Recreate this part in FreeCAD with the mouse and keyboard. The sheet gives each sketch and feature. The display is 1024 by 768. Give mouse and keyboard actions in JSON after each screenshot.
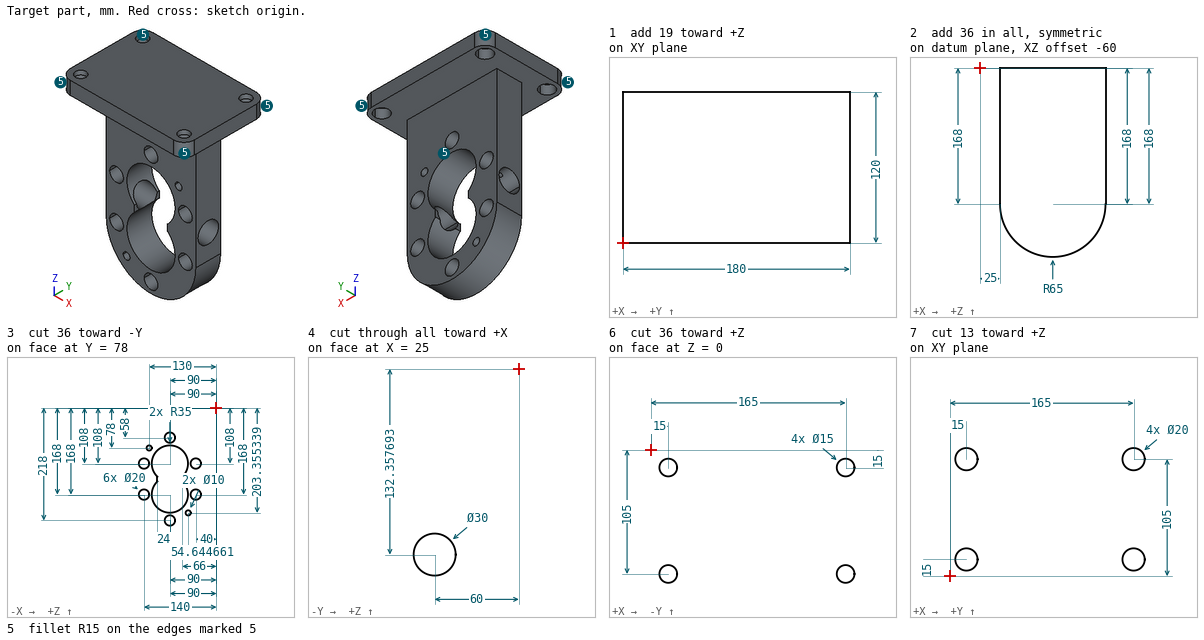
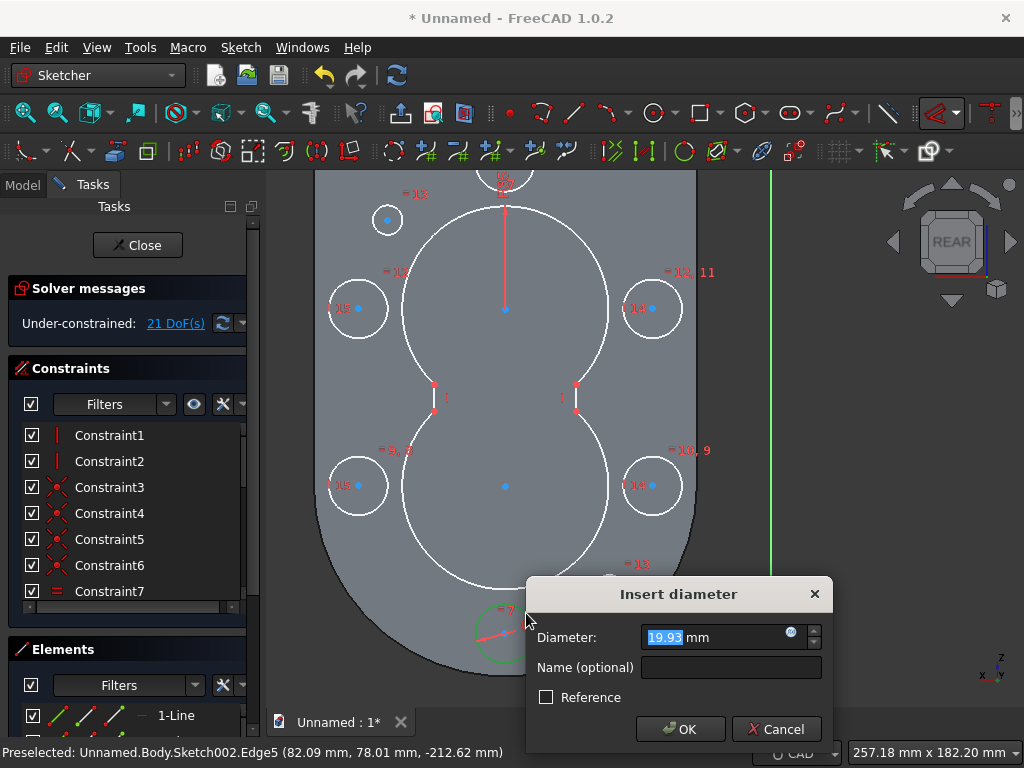
{"action": "type", "text": "20"}
{"action": "key", "text": "Return"}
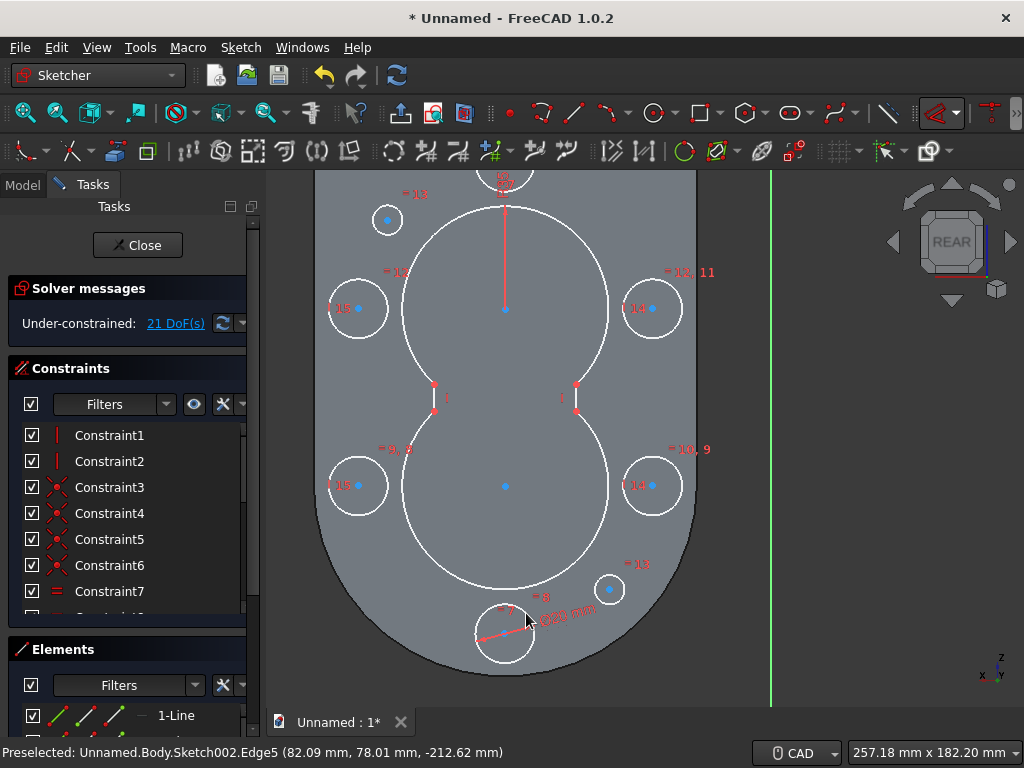
{"action": "scroll", "coordinate": [620, 579], "scroll_direction": "up", "scroll_amount": 2}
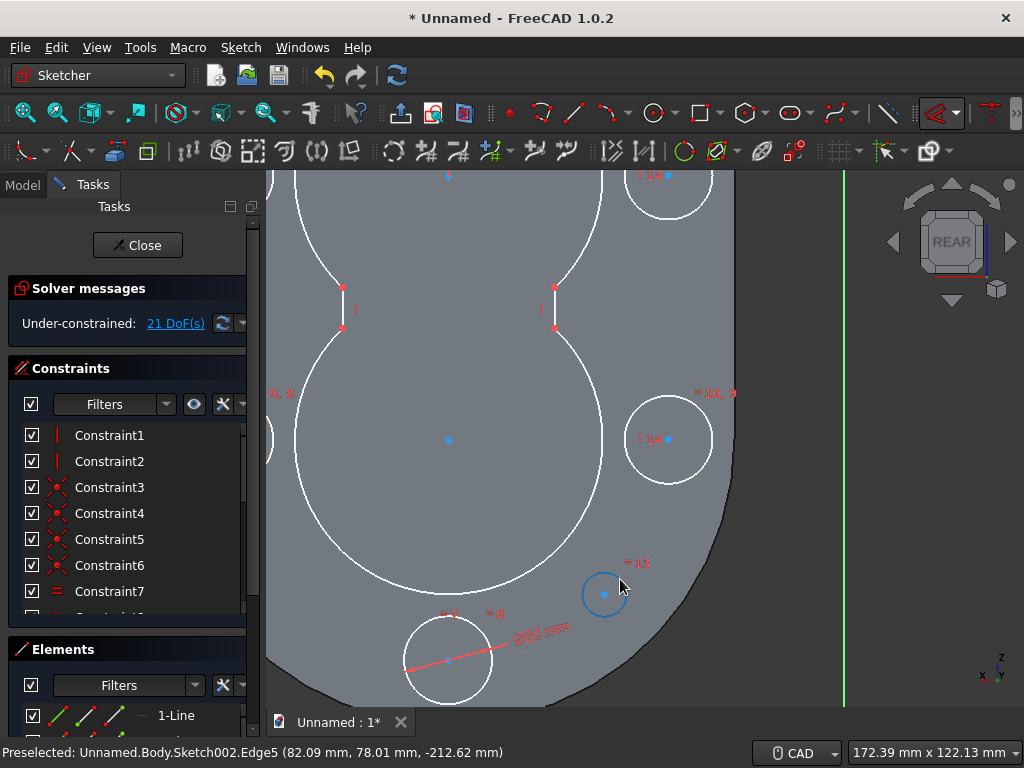
{"action": "left_click", "coordinate": [620, 579]}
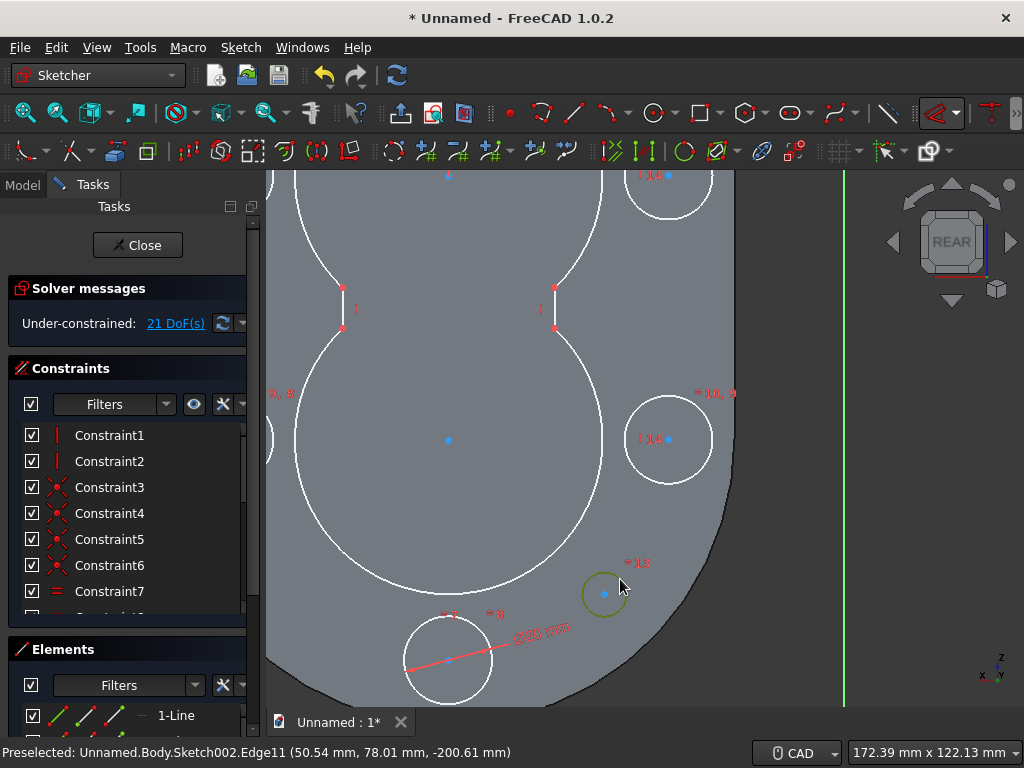
{"action": "left_click", "coordinate": [958, 114]}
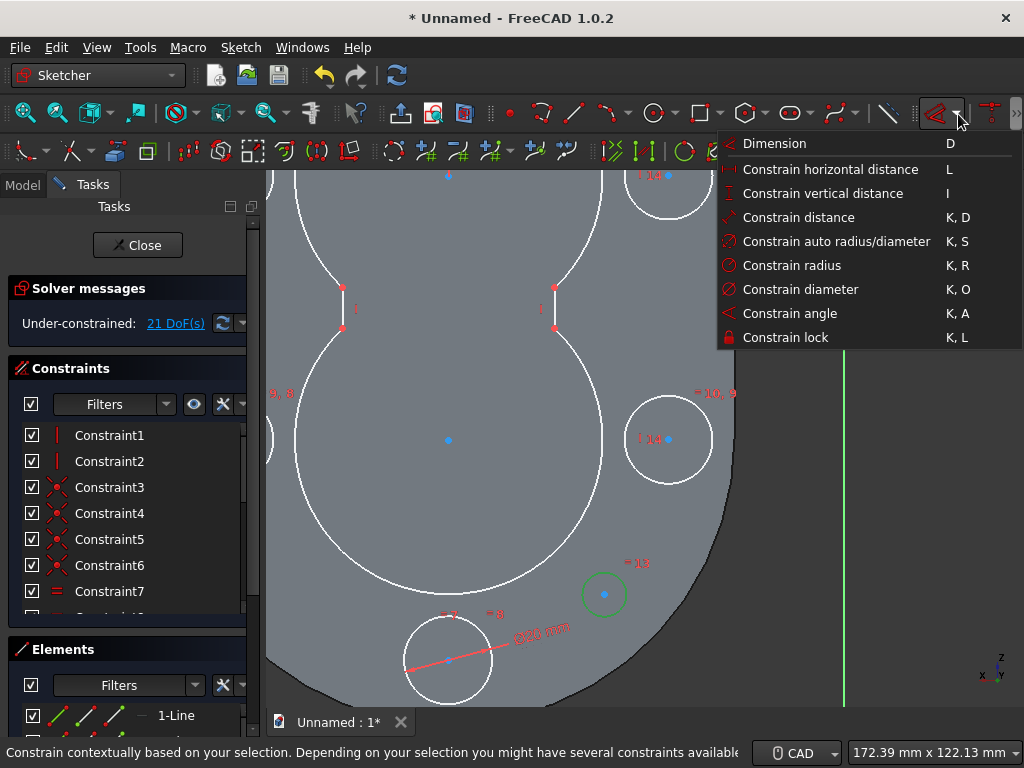
{"action": "left_click", "coordinate": [870, 289]}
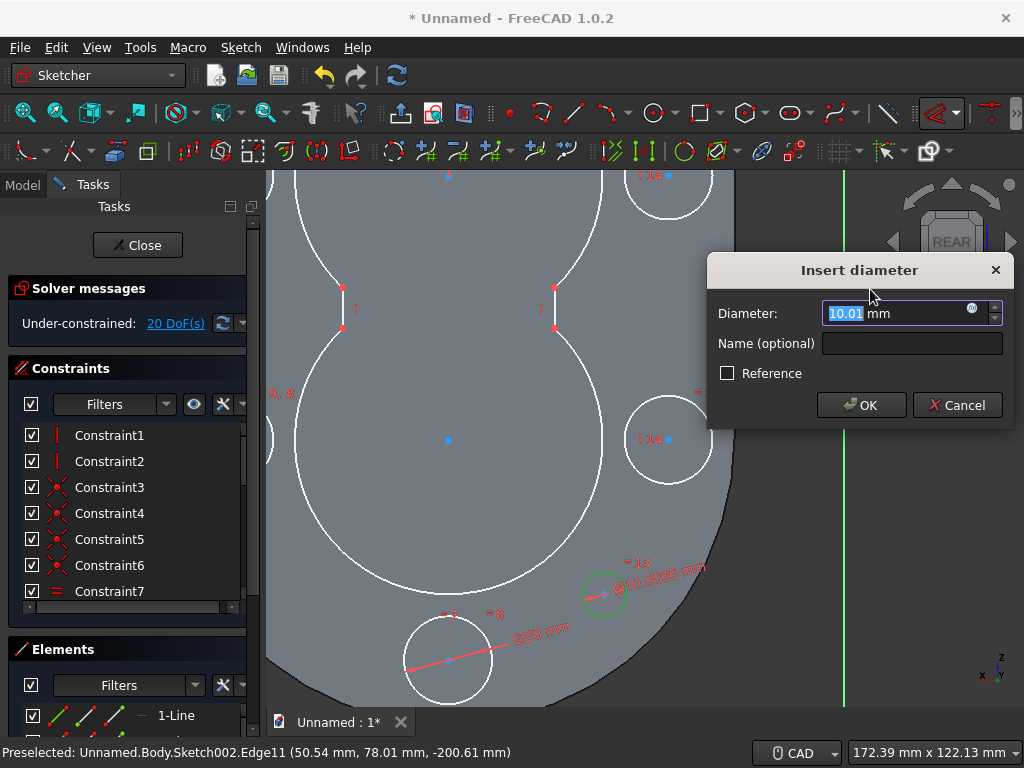
{"action": "type", "text": "10"}
{"action": "key", "text": "Return"}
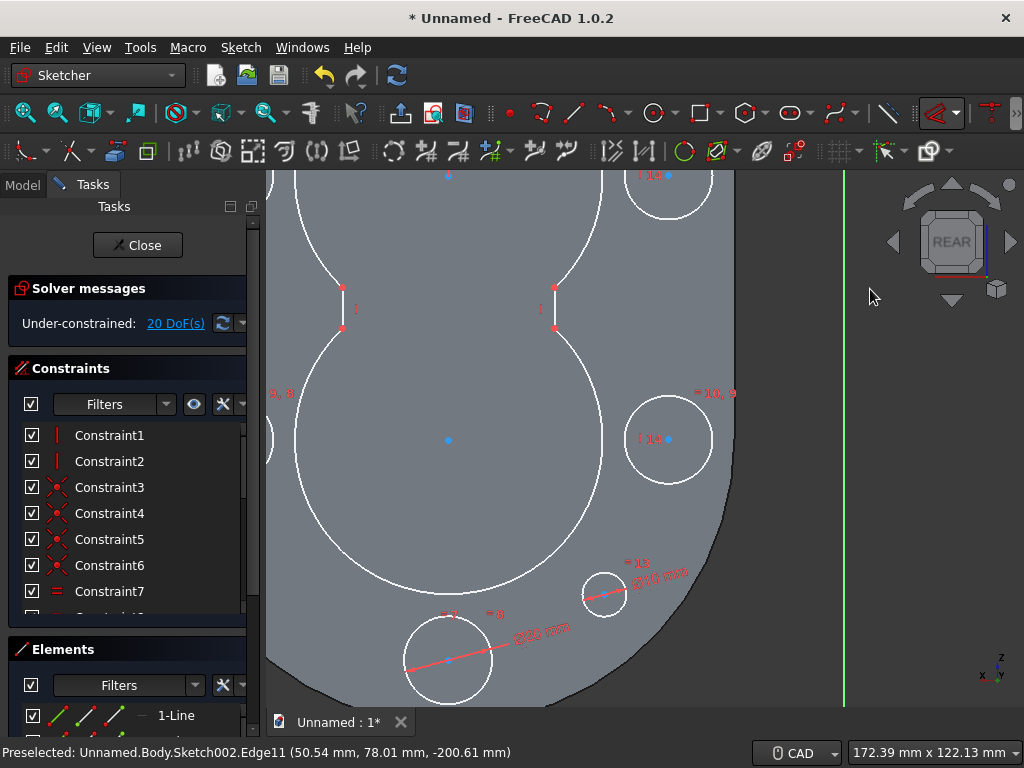
{"action": "left_click", "coordinate": [448, 660]}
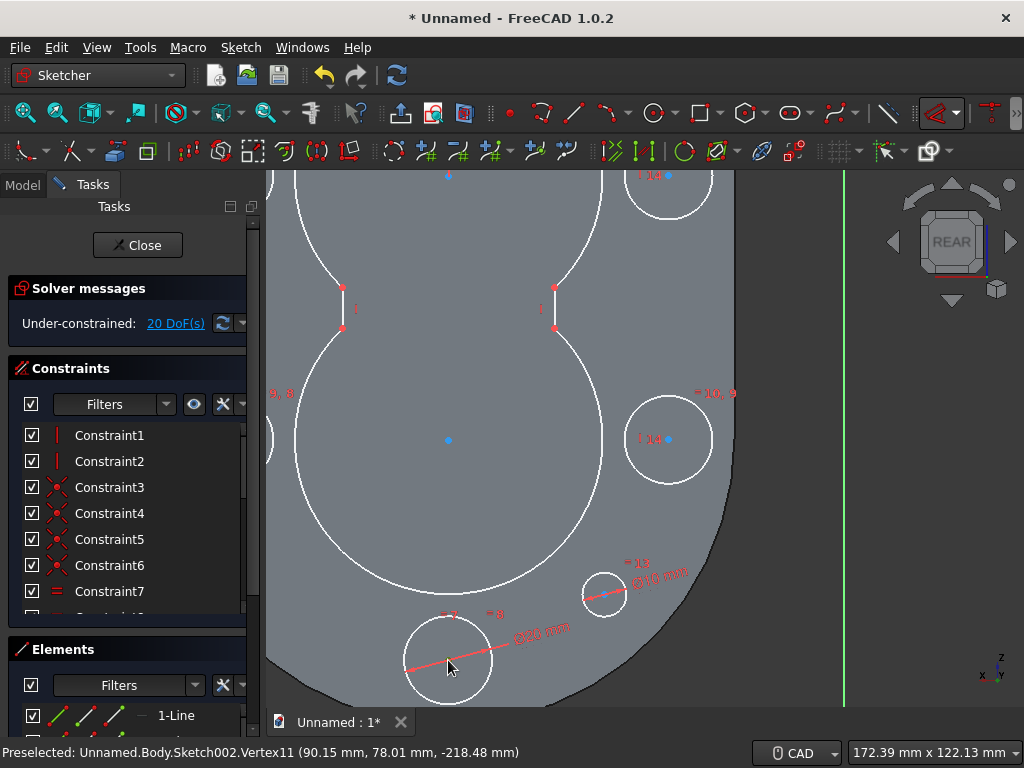
{"action": "left_click", "coordinate": [958, 114]}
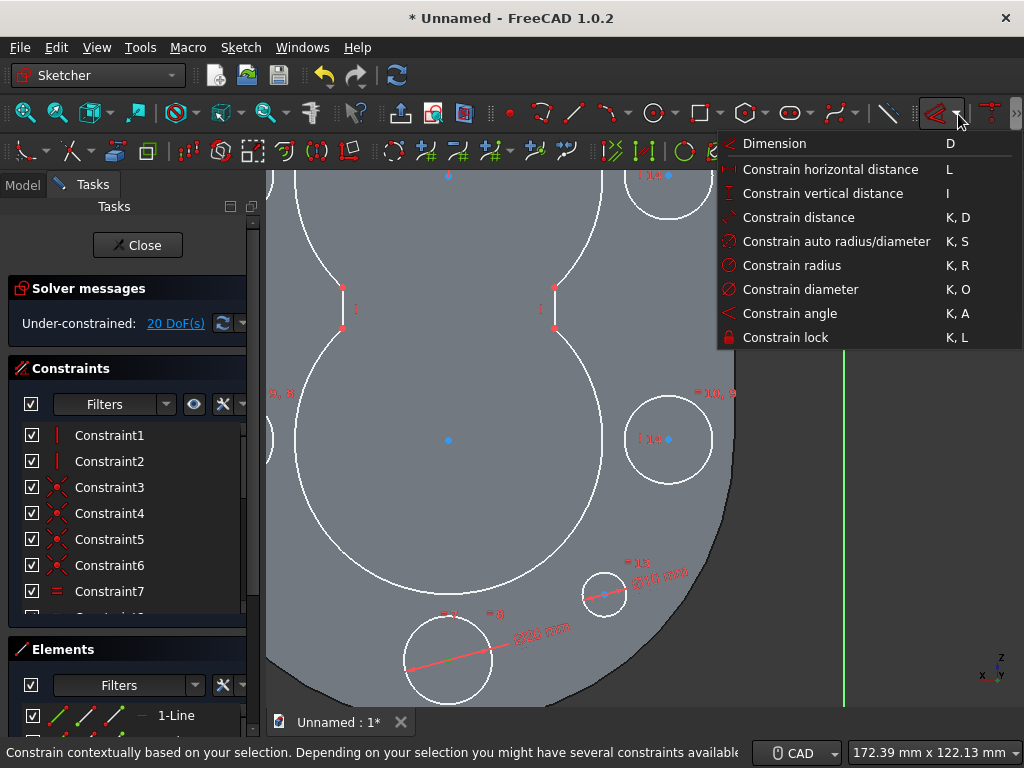
{"action": "left_click", "coordinate": [870, 169]}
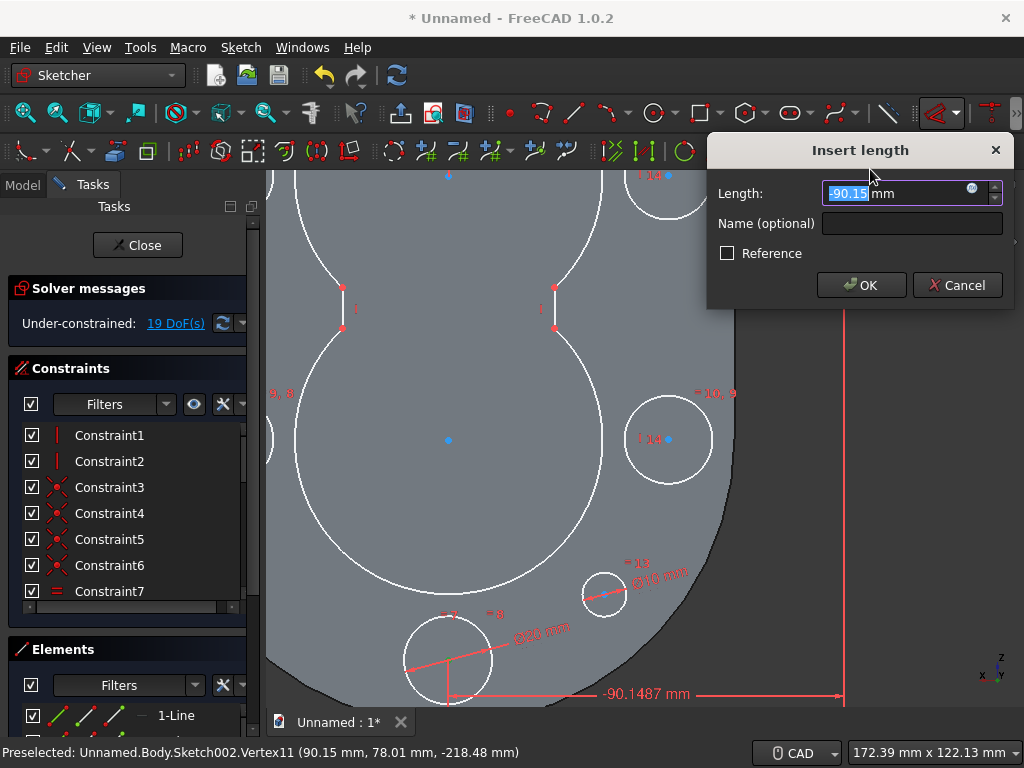
{"action": "type", "text": "-90"}
{"action": "key", "text": "Return"}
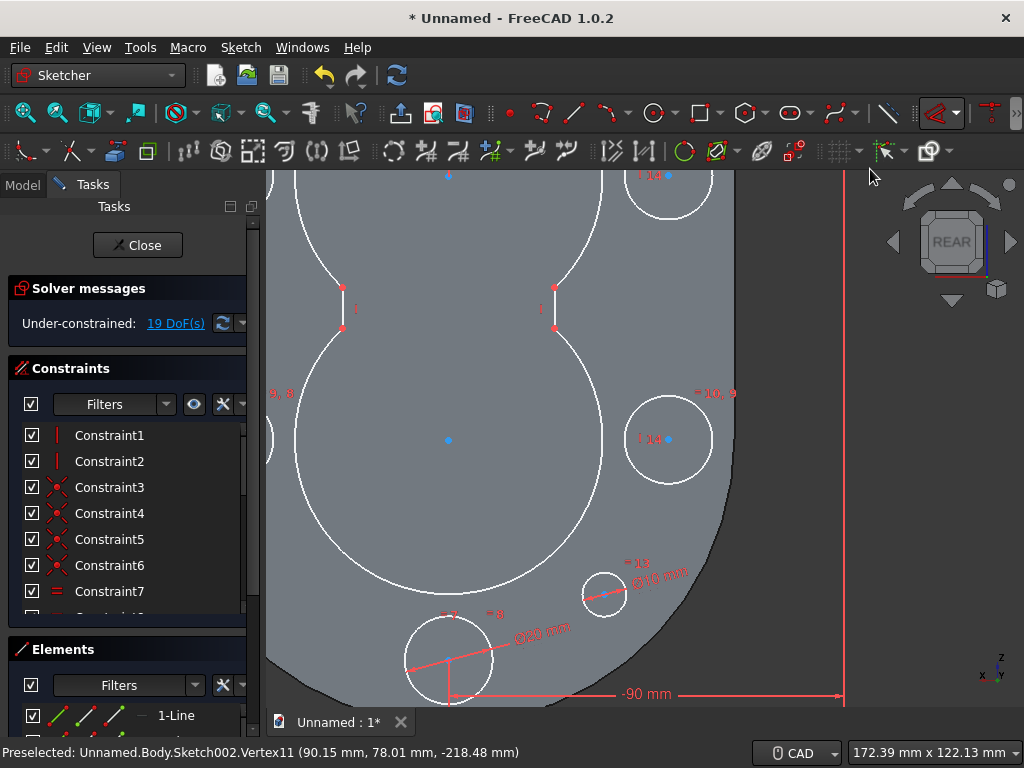
{"action": "left_click", "coordinate": [669, 440]}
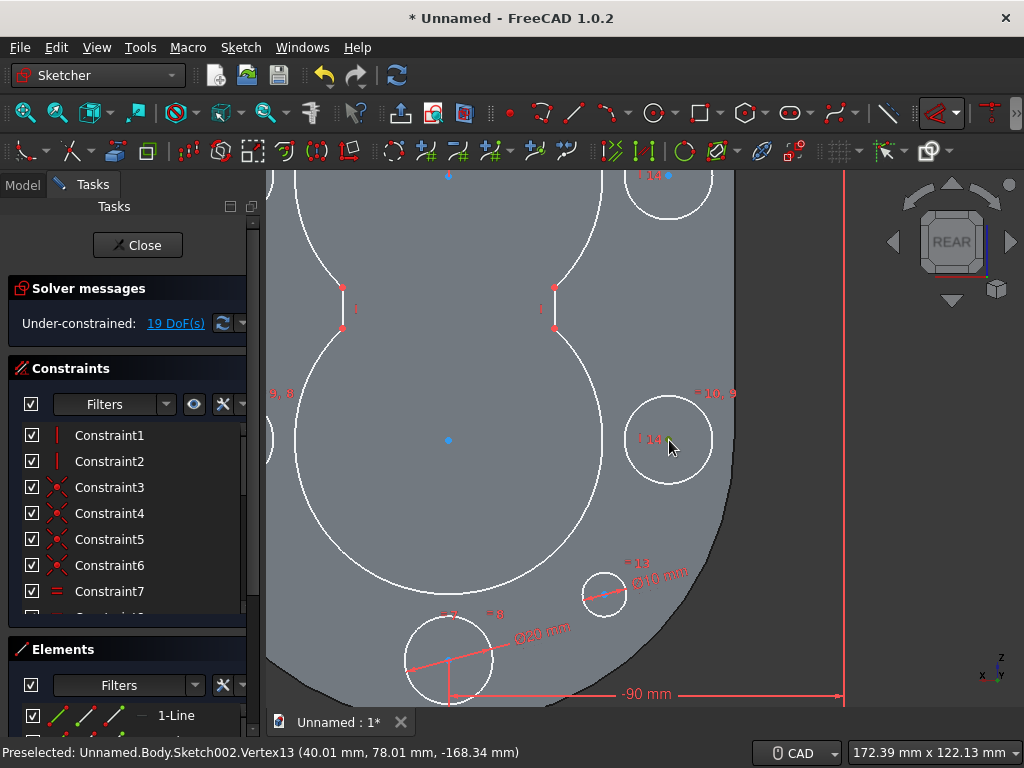
{"action": "key", "text": "l"}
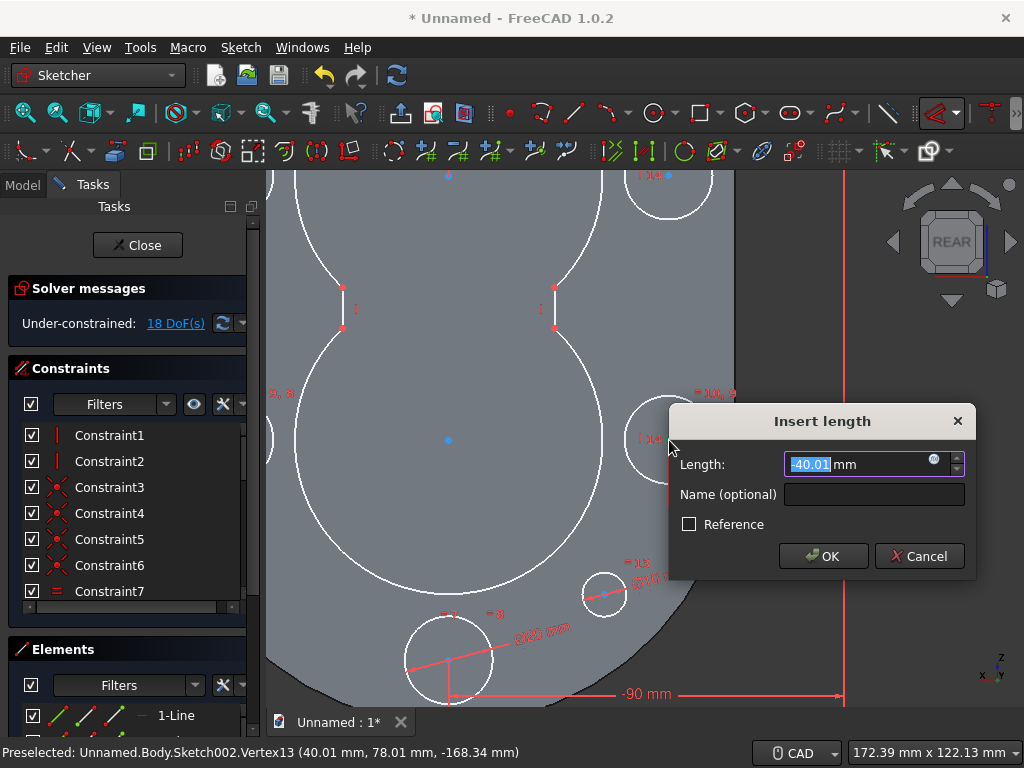
{"action": "type", "text": "-40"}
{"action": "key", "text": "Return"}